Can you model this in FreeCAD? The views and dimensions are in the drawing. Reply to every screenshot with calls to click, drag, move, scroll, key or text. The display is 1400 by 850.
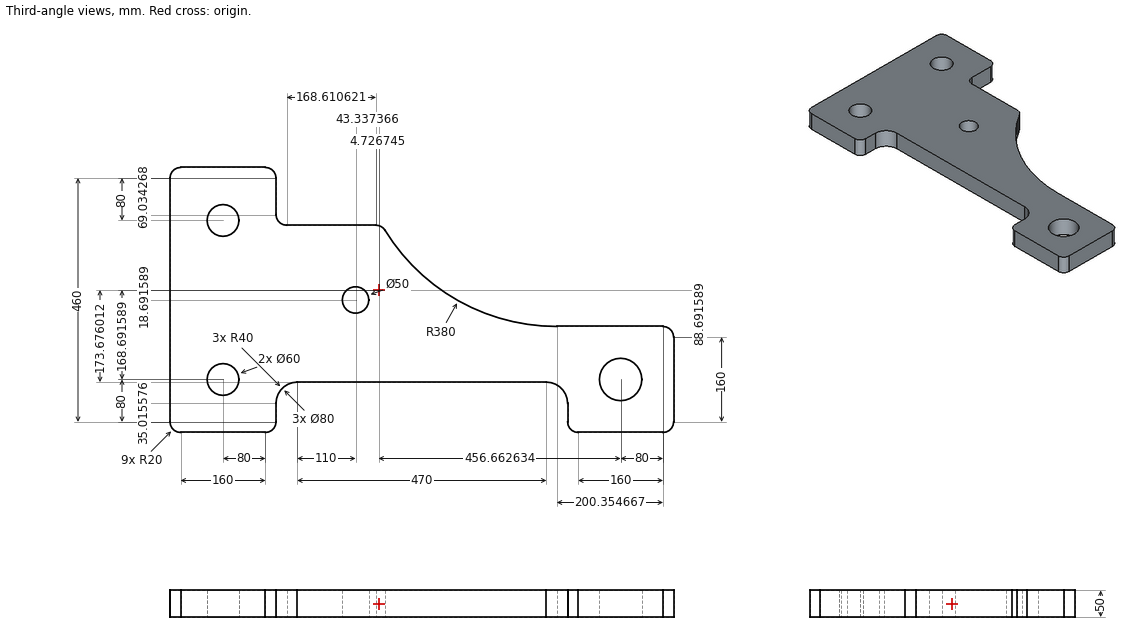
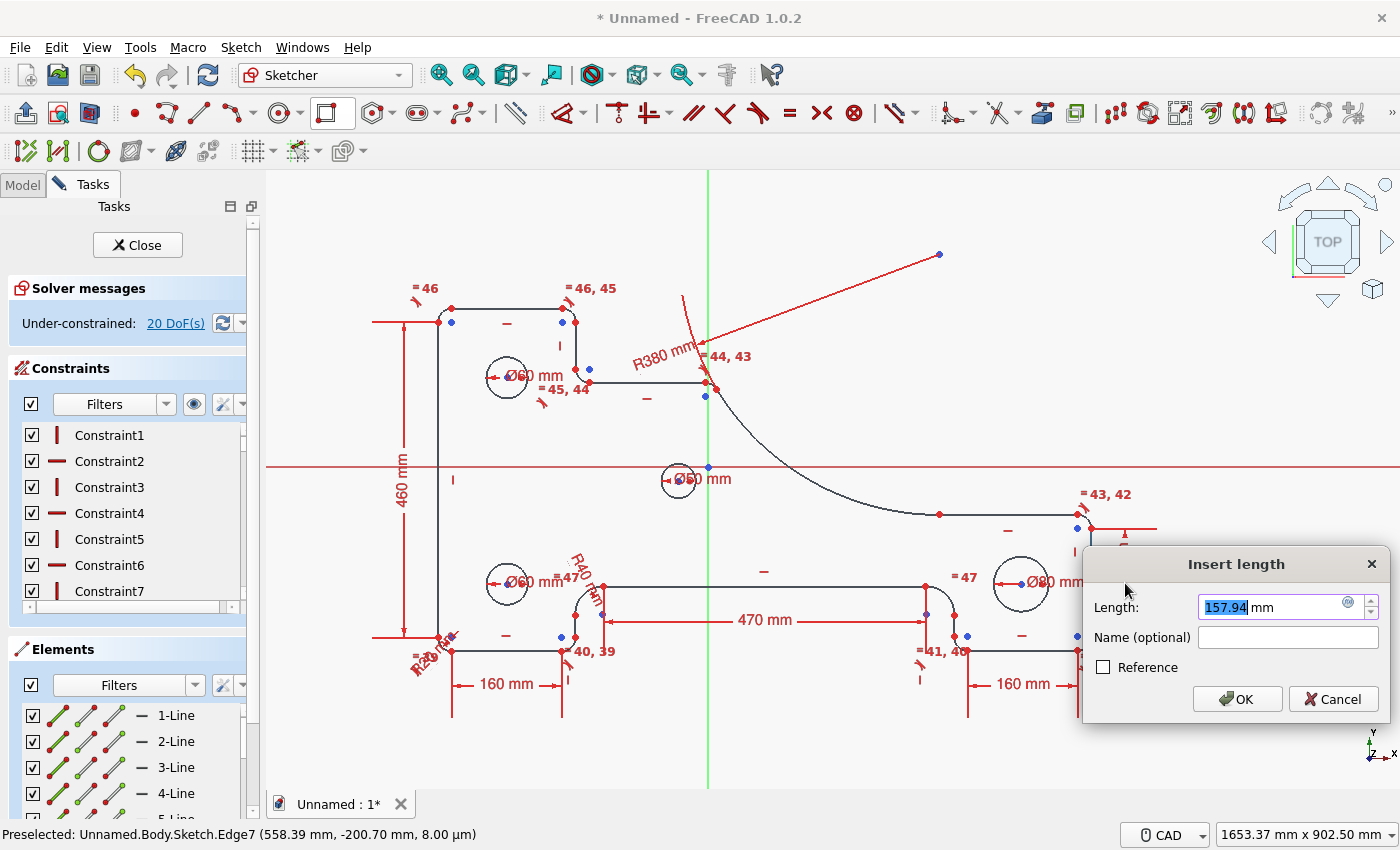
text(160)
key(Return)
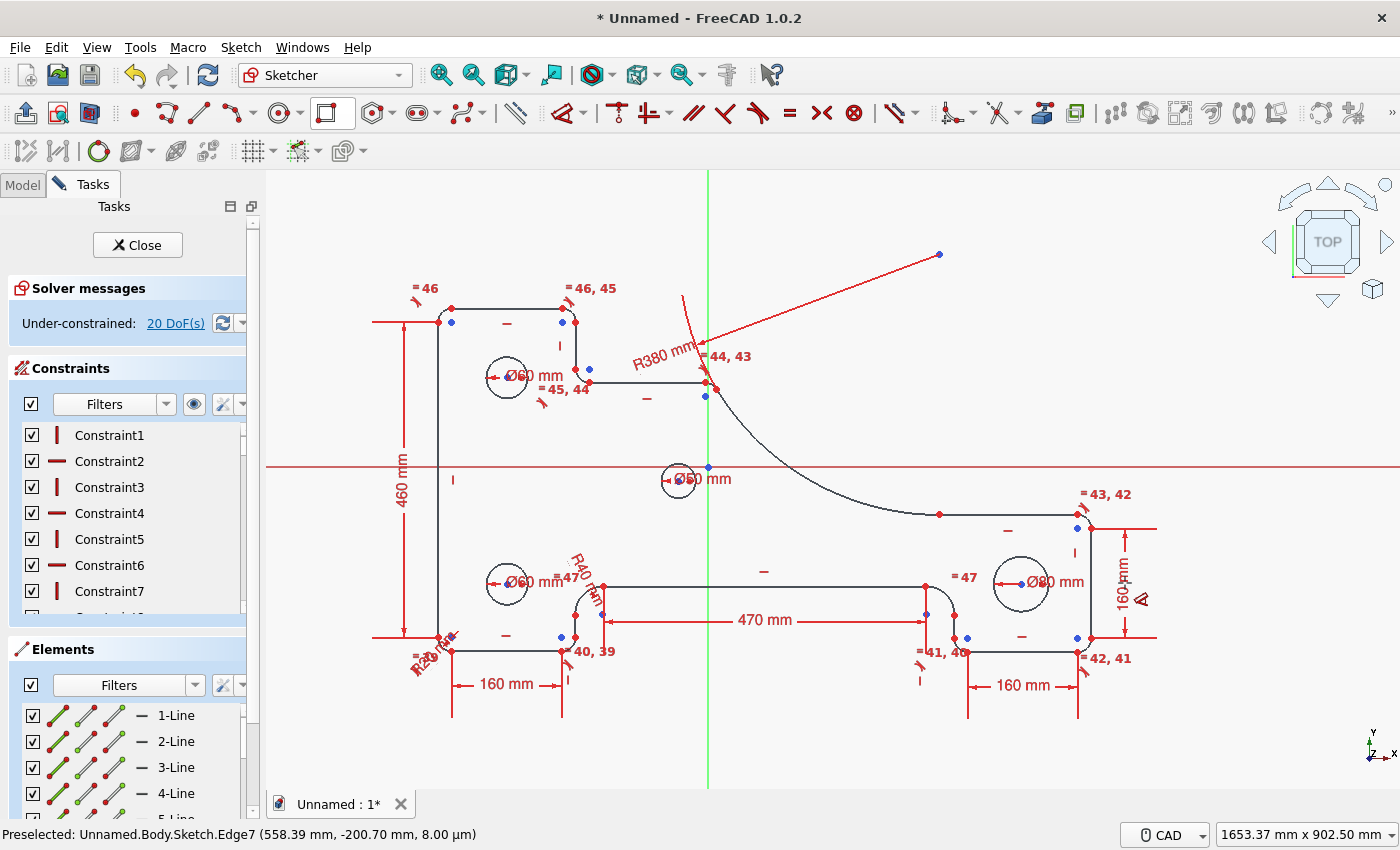
click(529, 309)
click(507, 275)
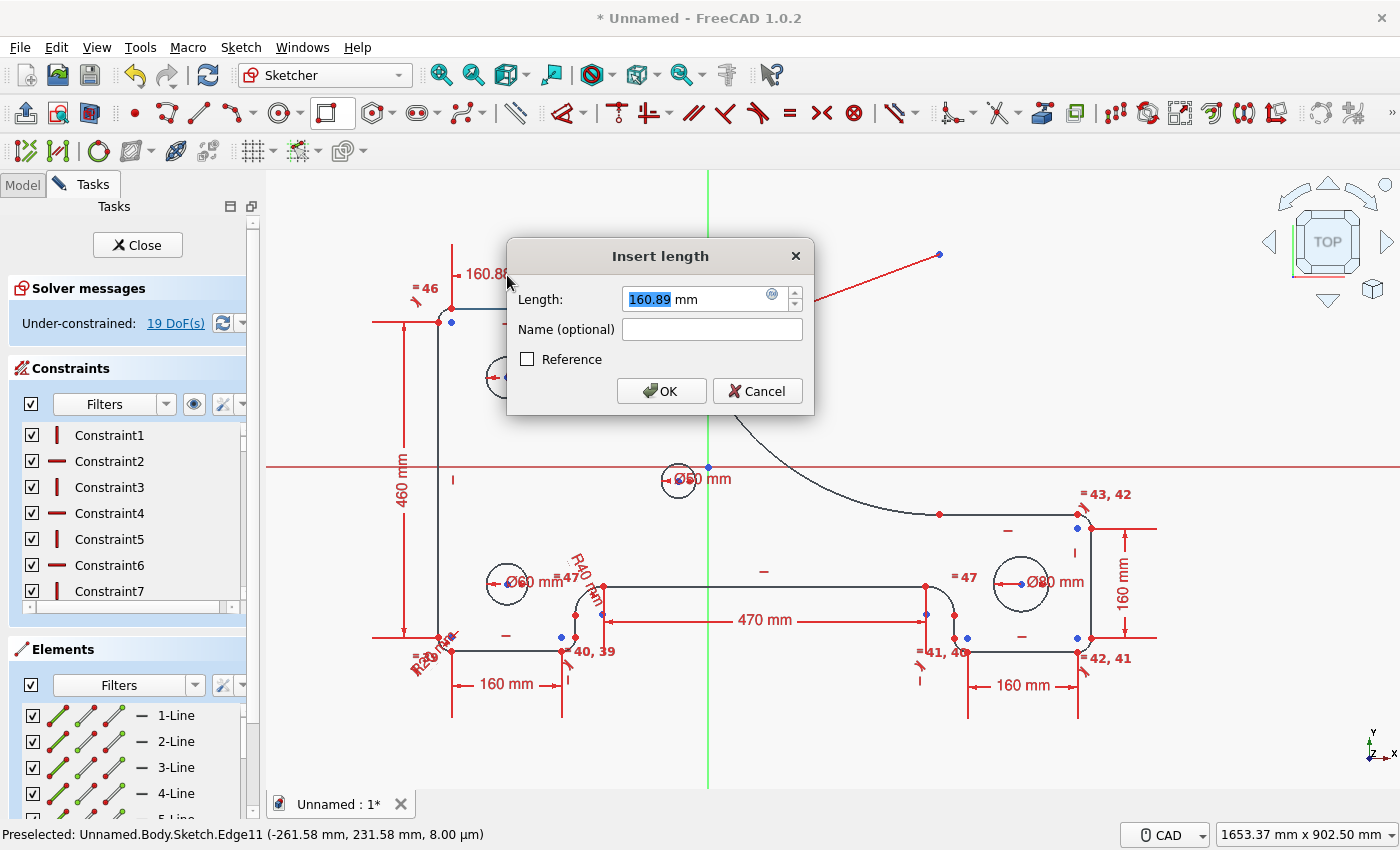
text(160)
key(Return)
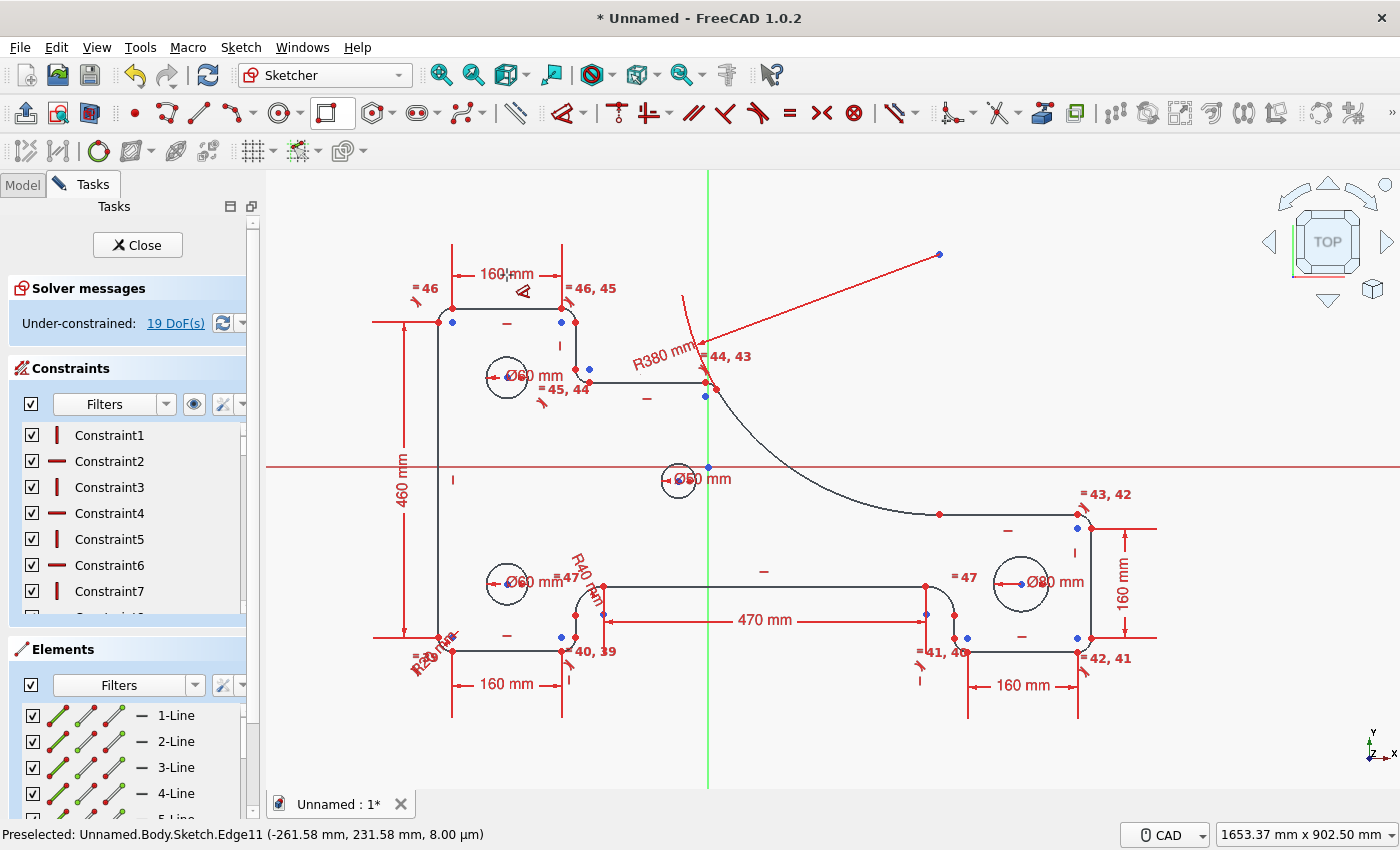
click(562, 651)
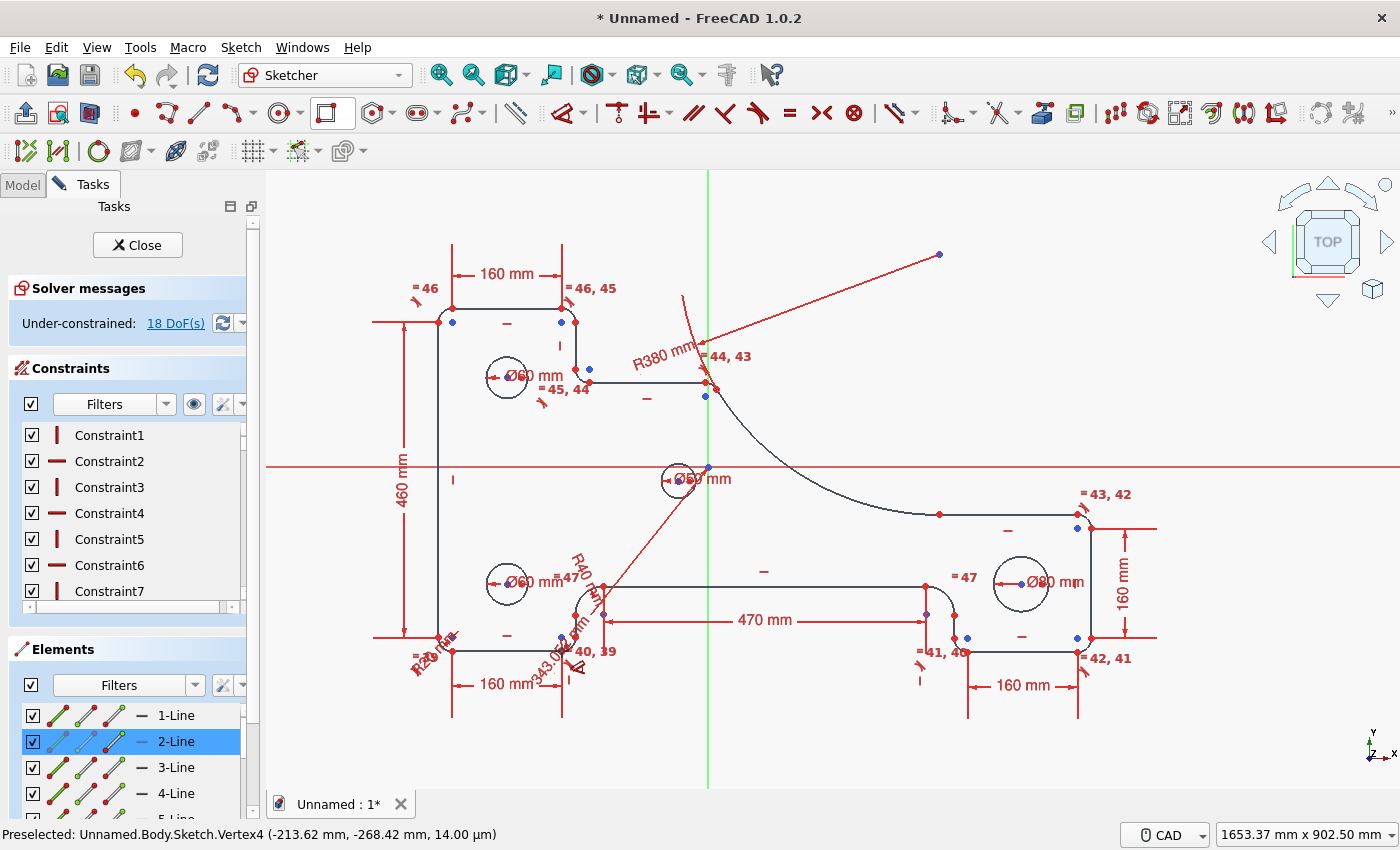
click(507, 584)
click(535, 550)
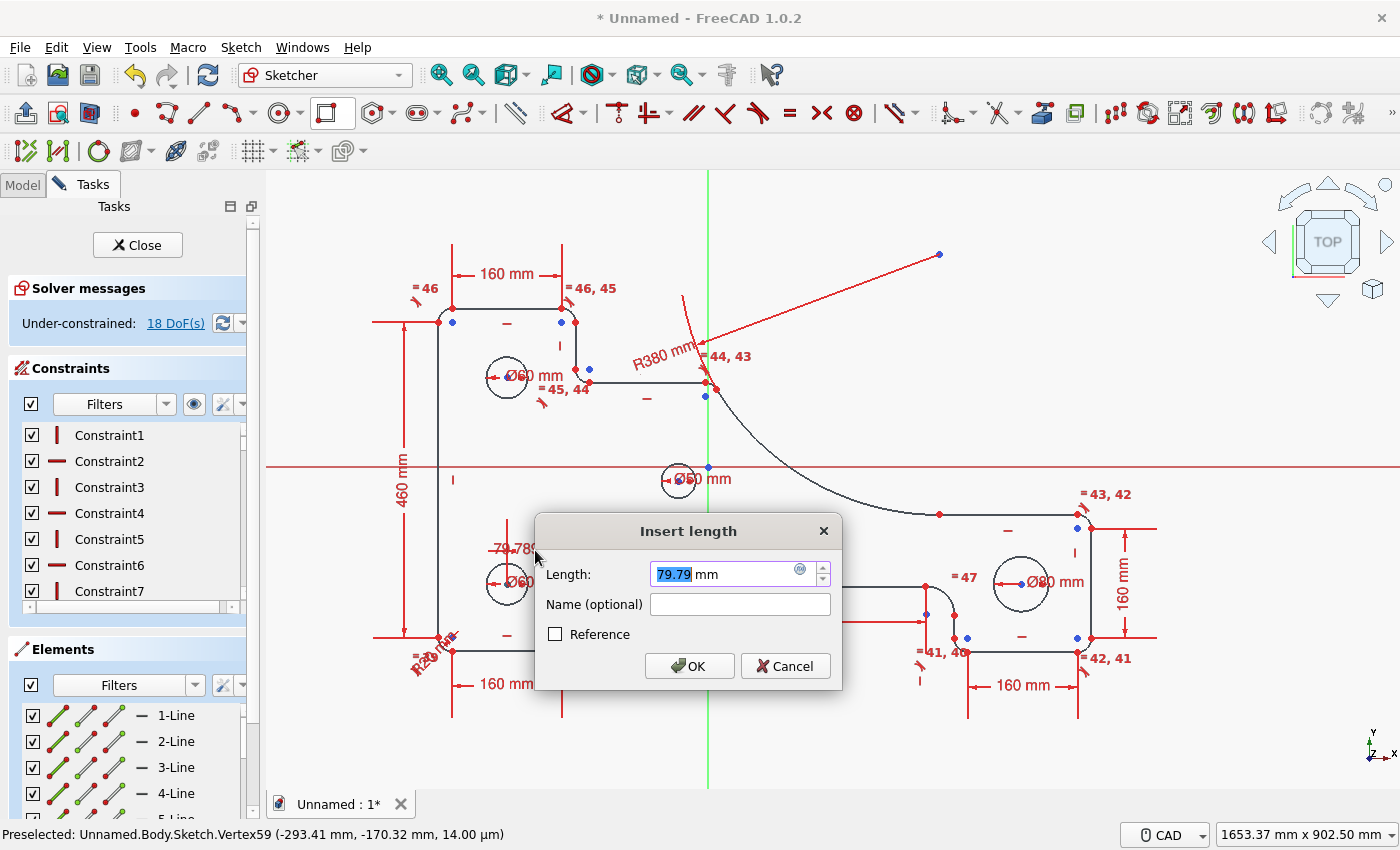
text(80)
key(Return)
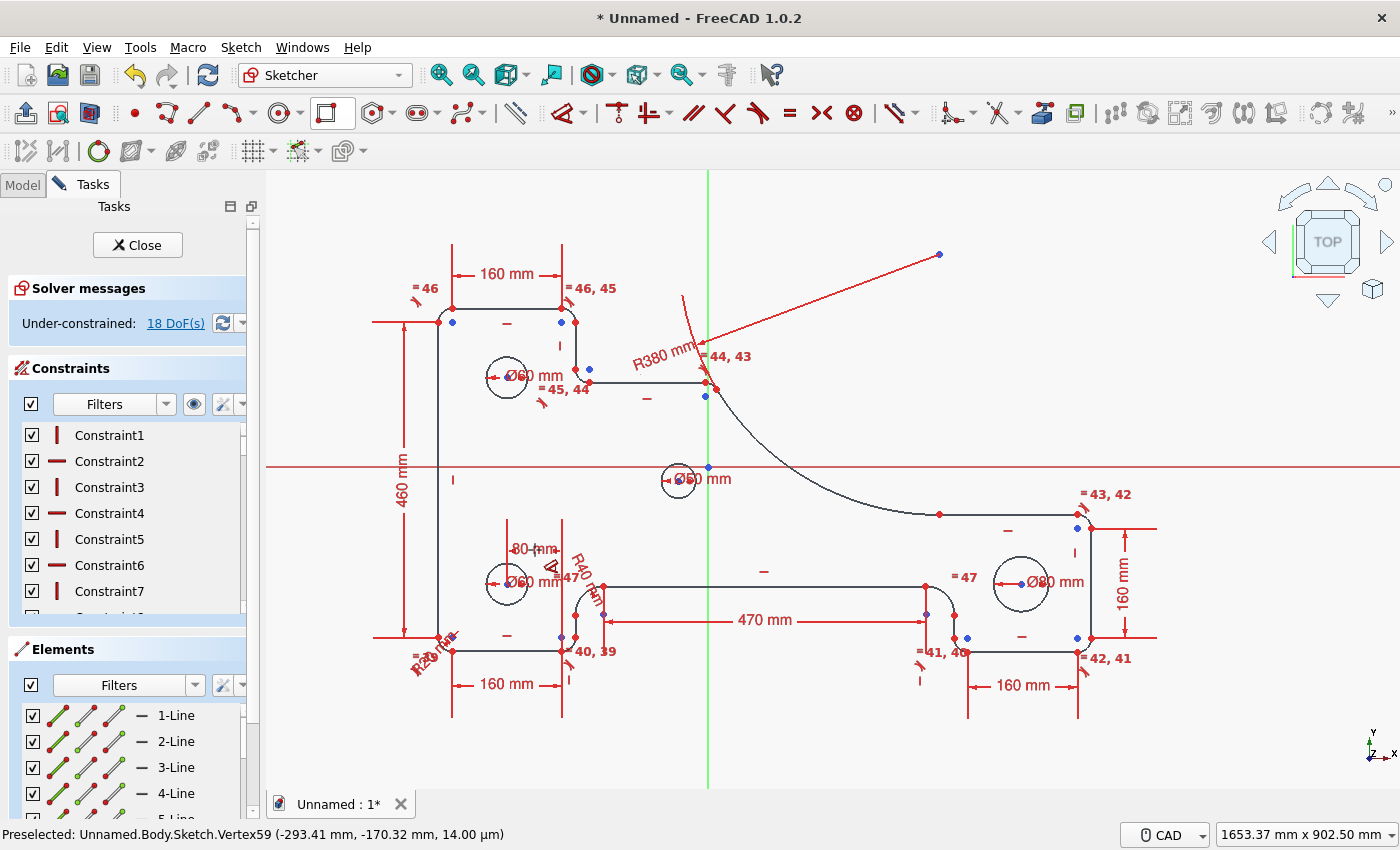
click(576, 638)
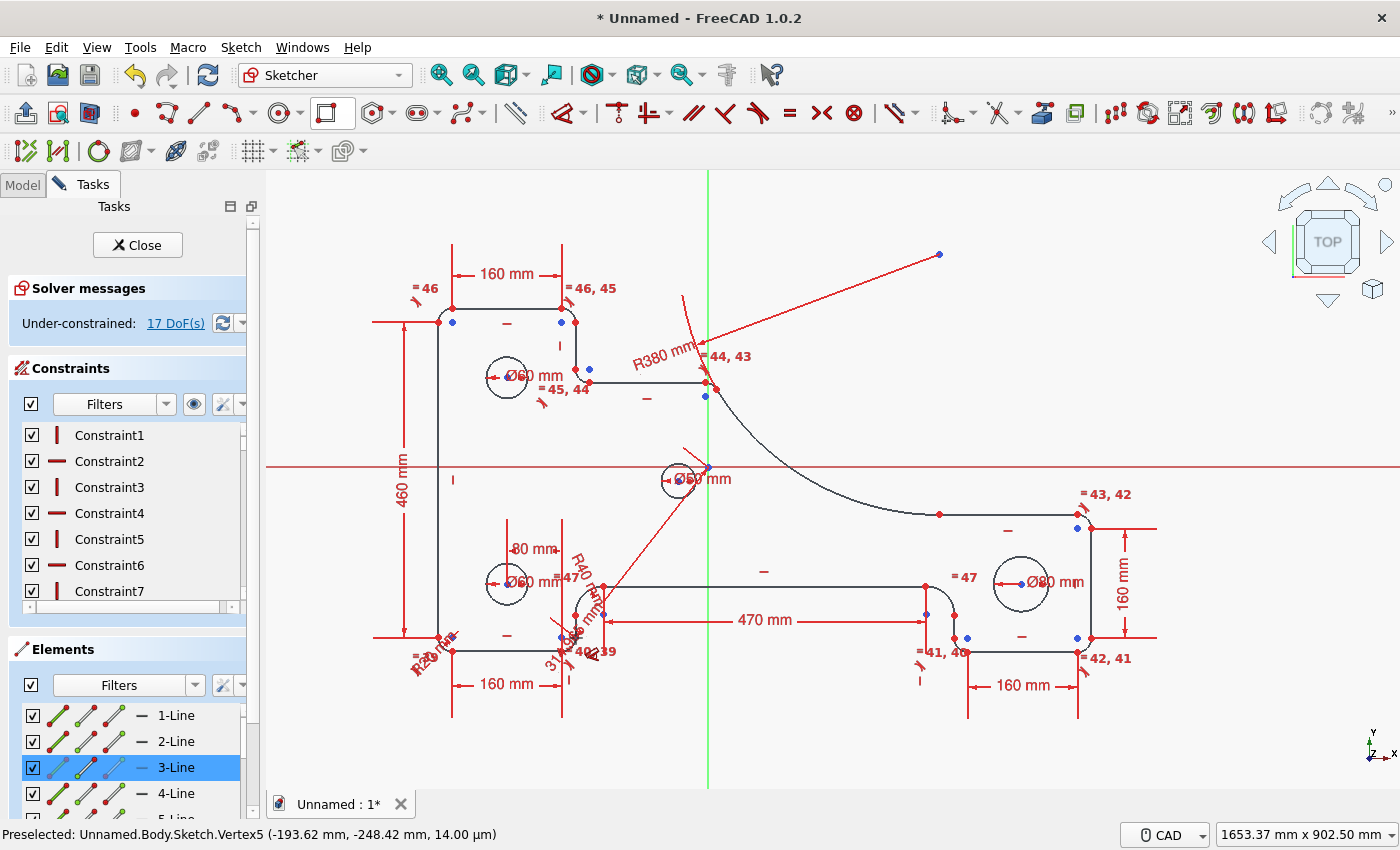
click(507, 584)
click(473, 611)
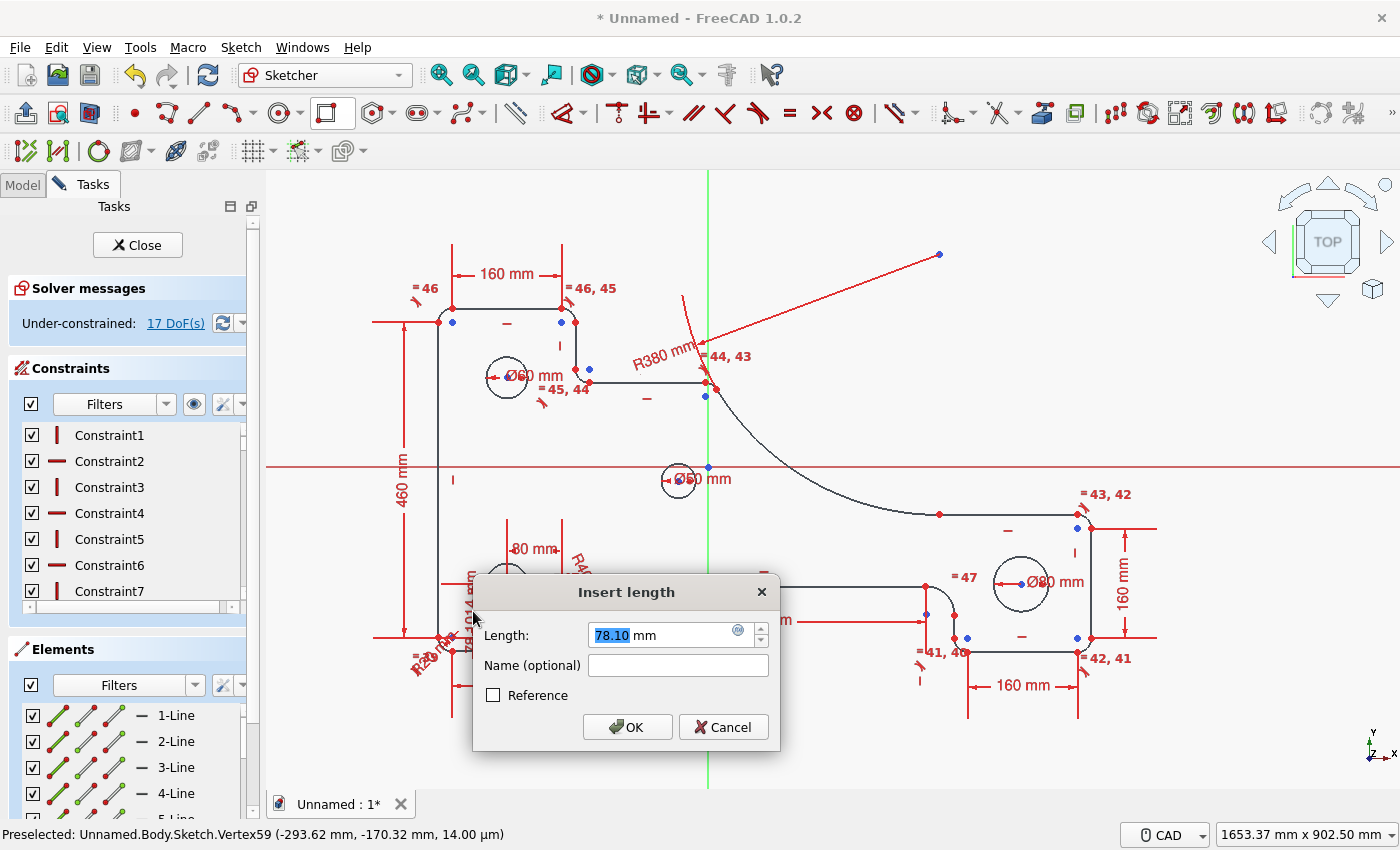
text(80)
key(Return)